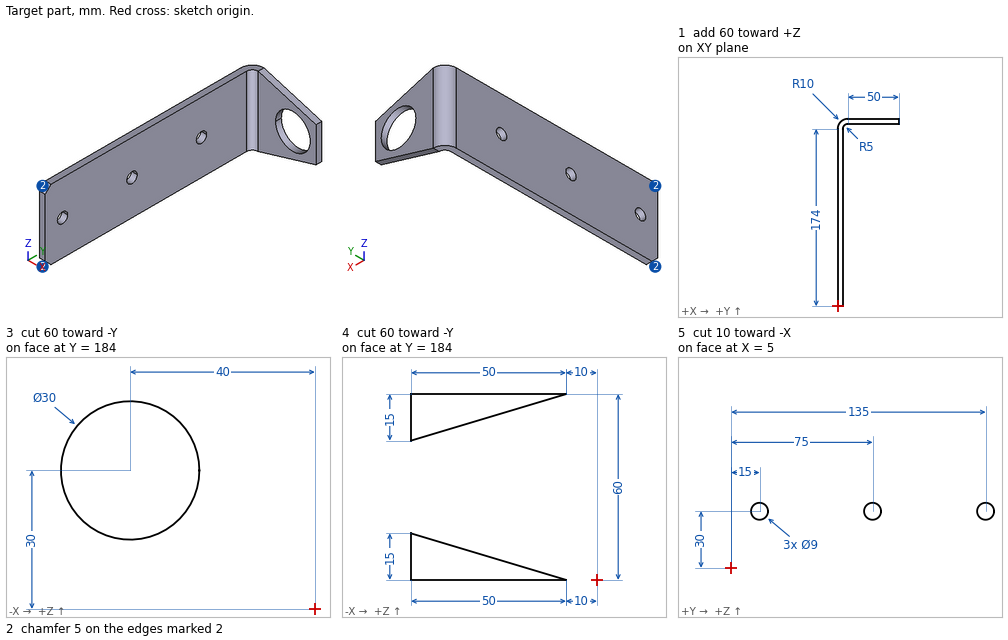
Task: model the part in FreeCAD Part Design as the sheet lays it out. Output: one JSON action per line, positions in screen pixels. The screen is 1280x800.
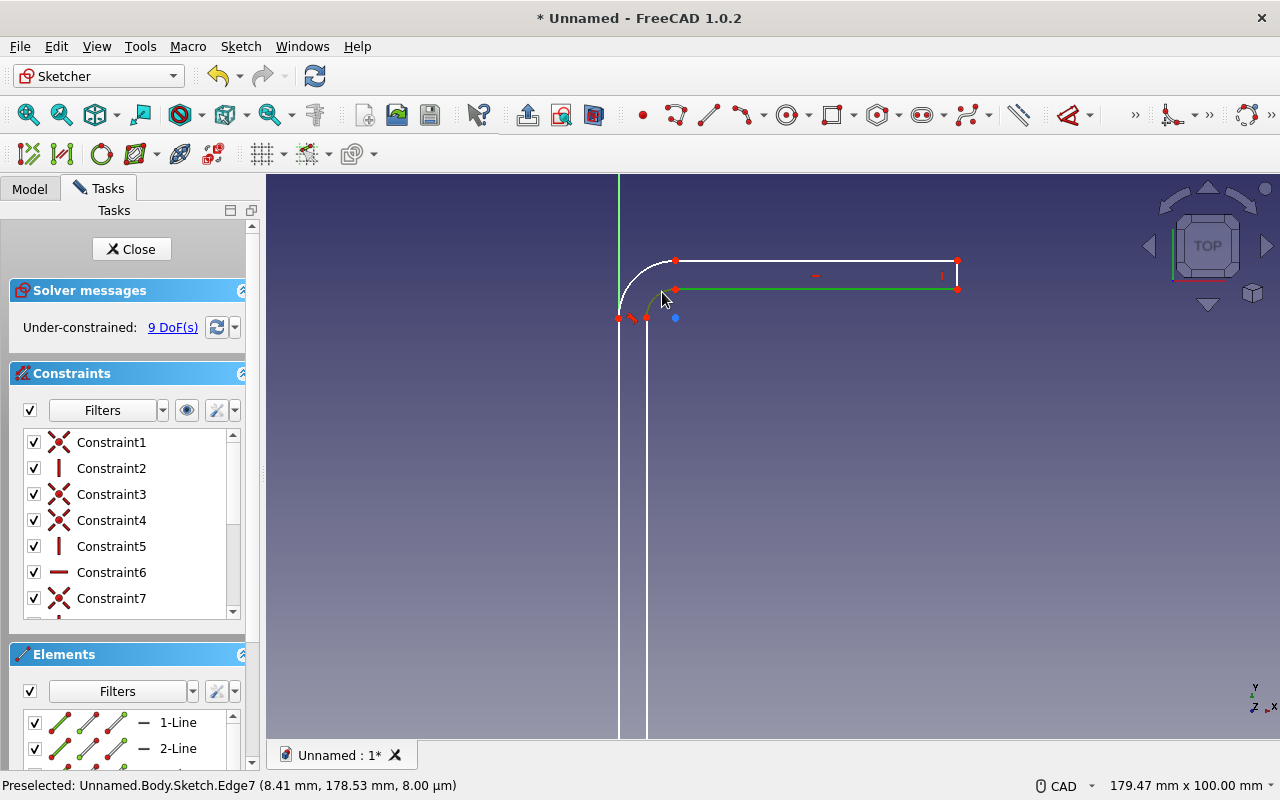
{"action": "key", "text": "t"}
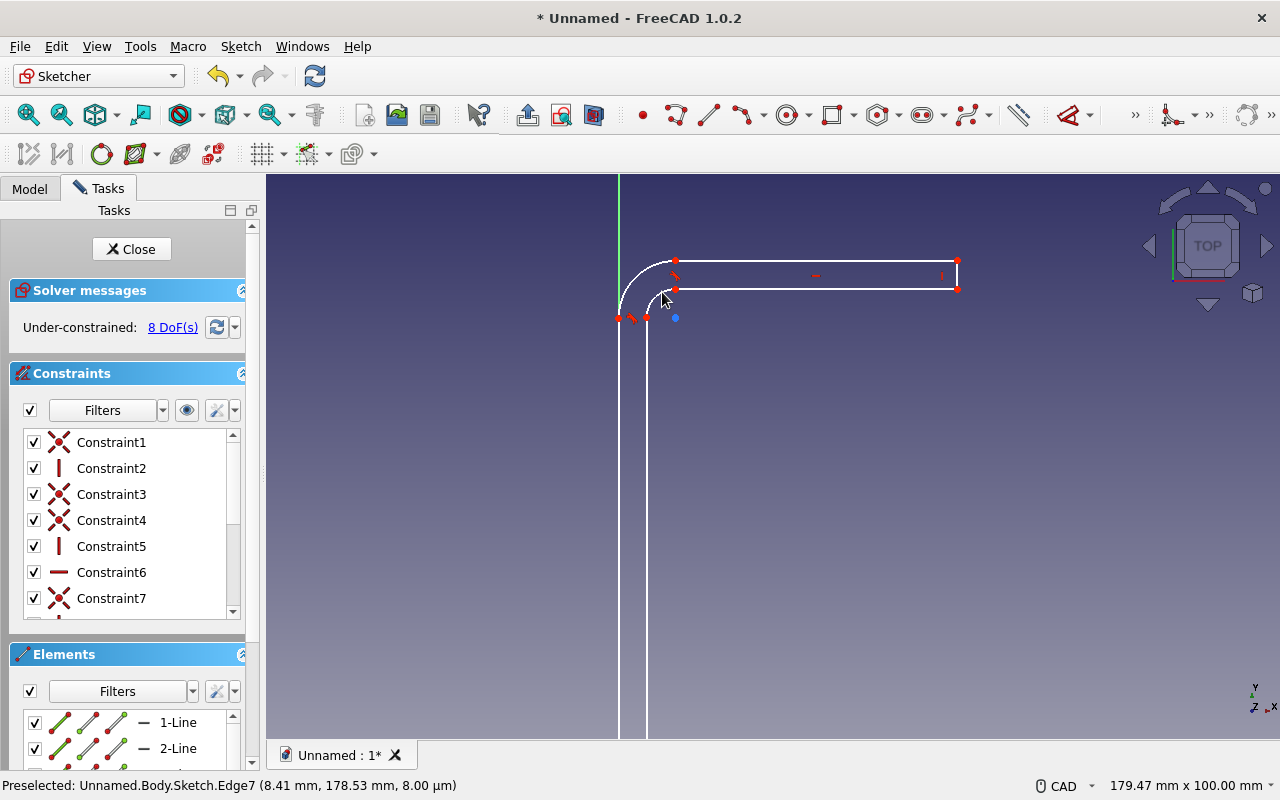
{"action": "left_click", "coordinate": [872, 261]}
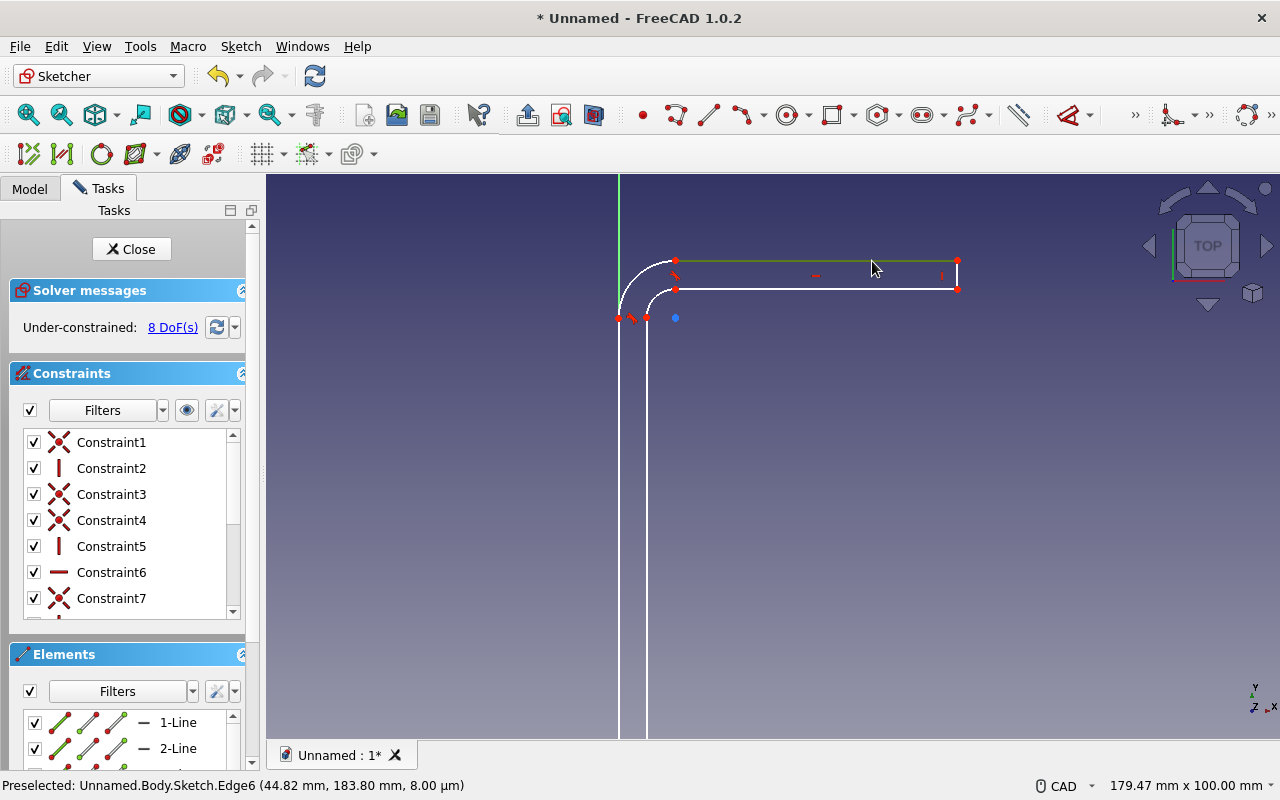
{"action": "left_click", "coordinate": [649, 267]}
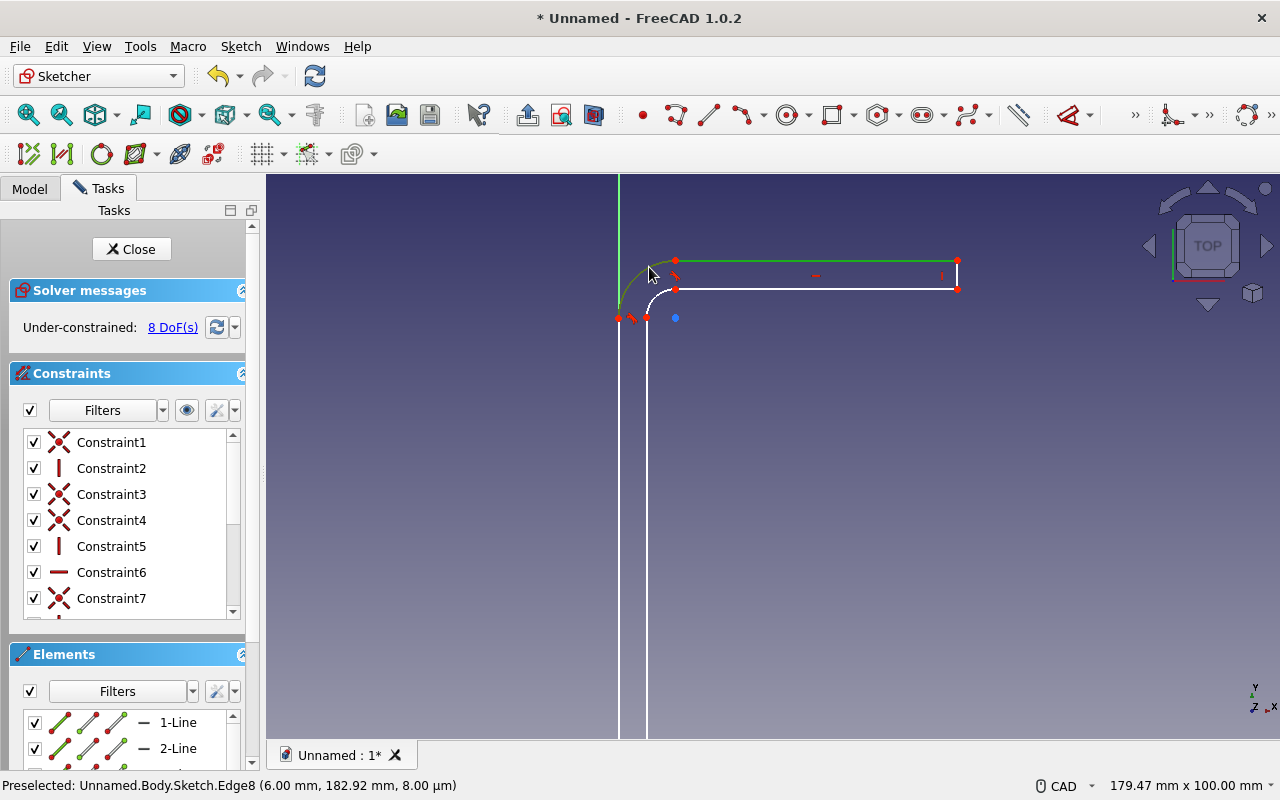
{"action": "key", "text": "t"}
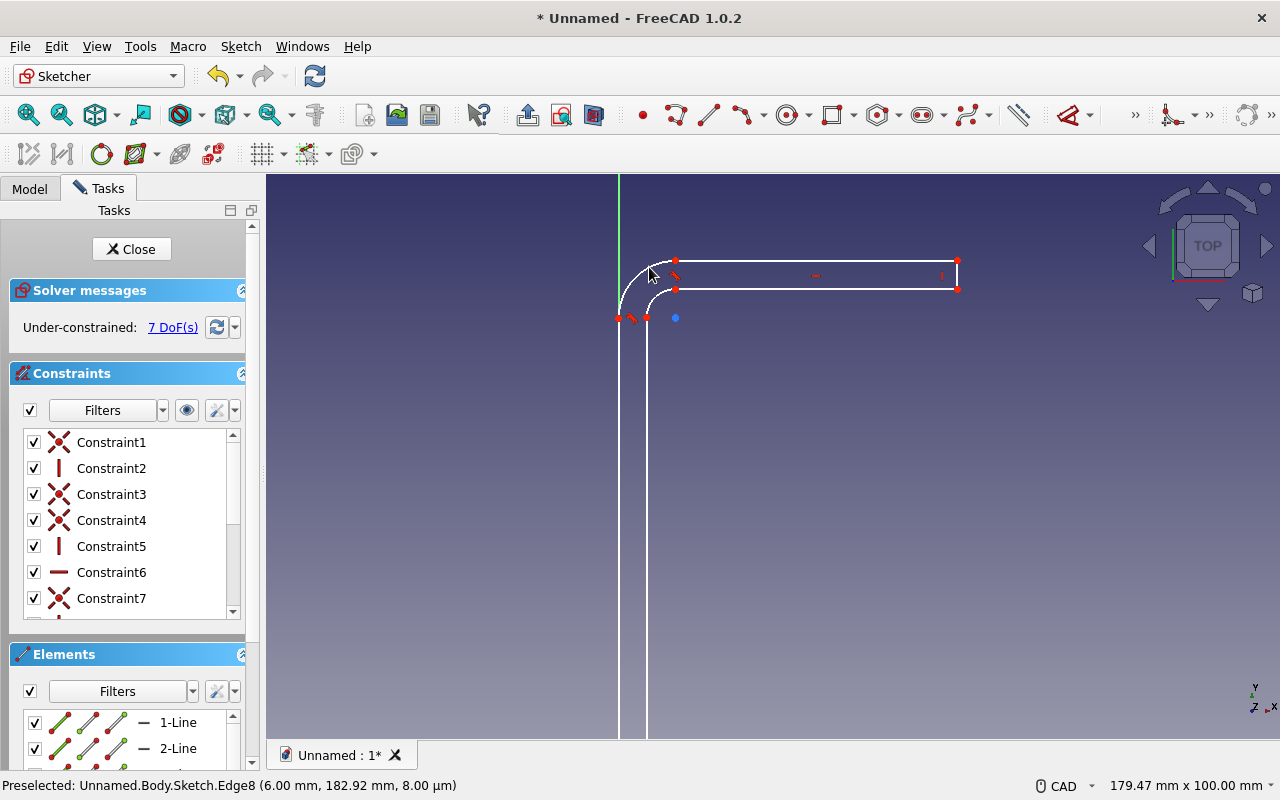
{"action": "scroll", "coordinate": [656, 269], "scroll_direction": "down", "scroll_amount": 5}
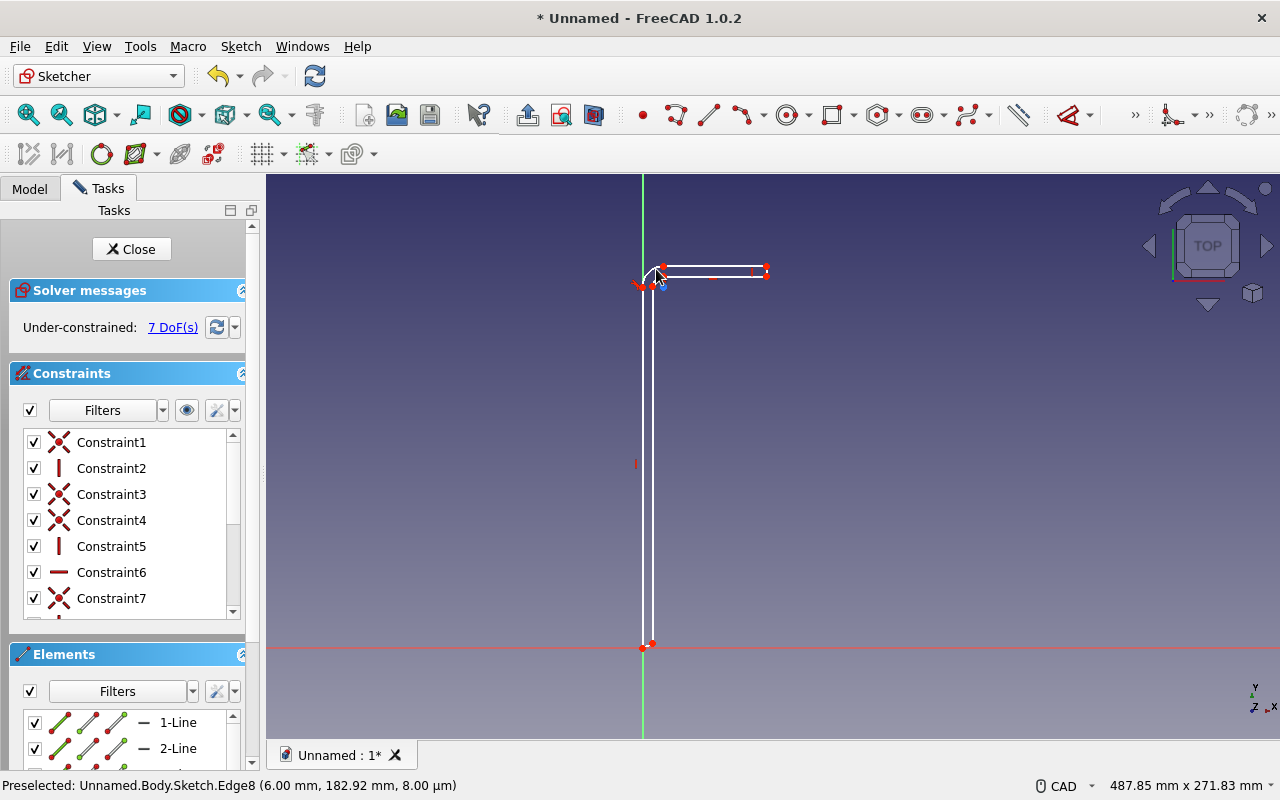
{"action": "scroll", "coordinate": [650, 645], "scroll_direction": "up", "scroll_amount": 8}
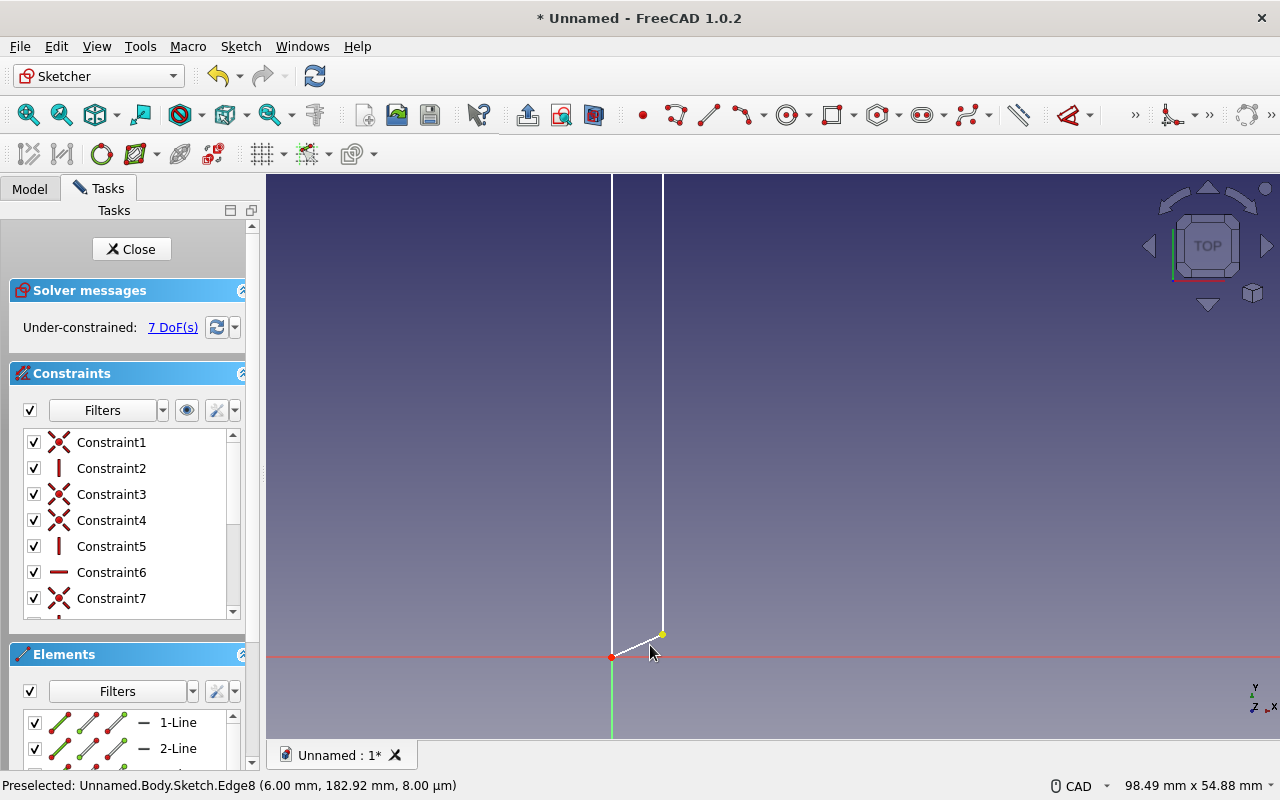
{"action": "left_click", "coordinate": [647, 641]}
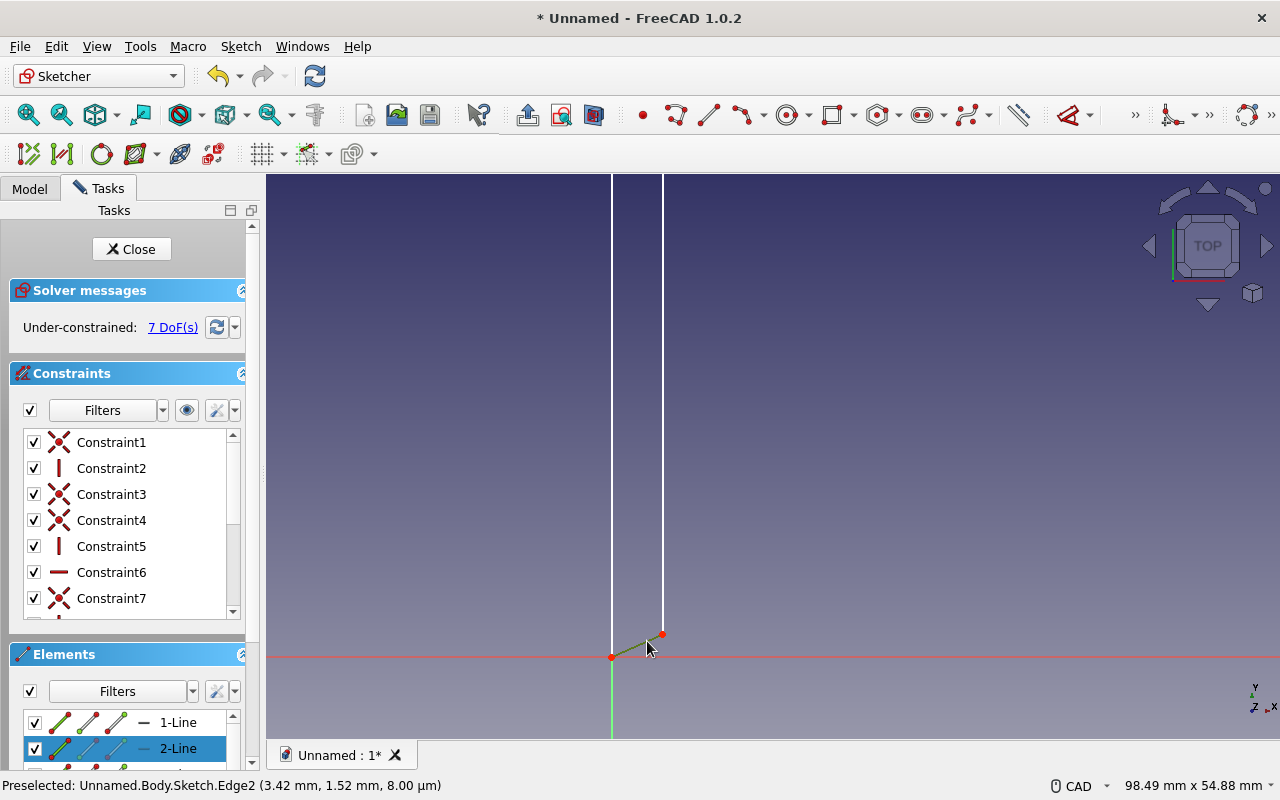
{"action": "key", "text": "h"}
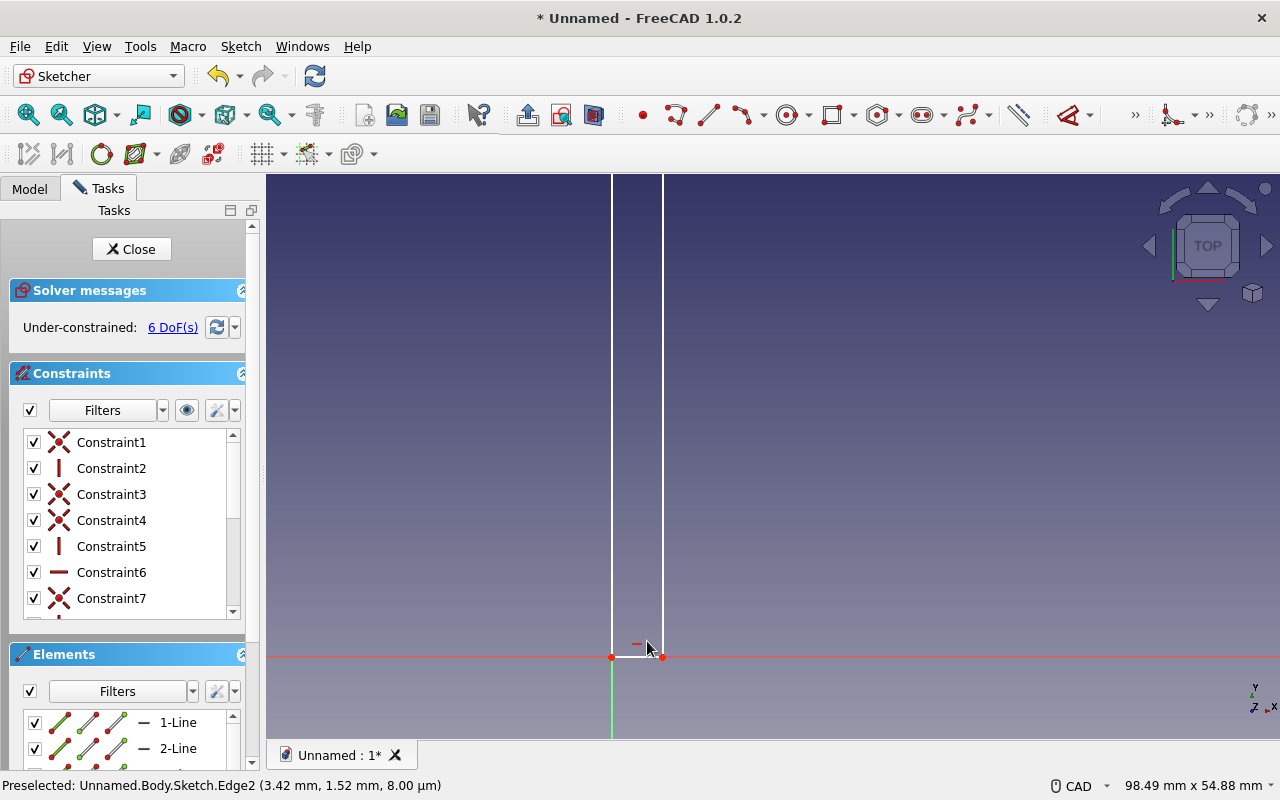
{"action": "scroll", "coordinate": [650, 645], "scroll_direction": "down", "scroll_amount": 8}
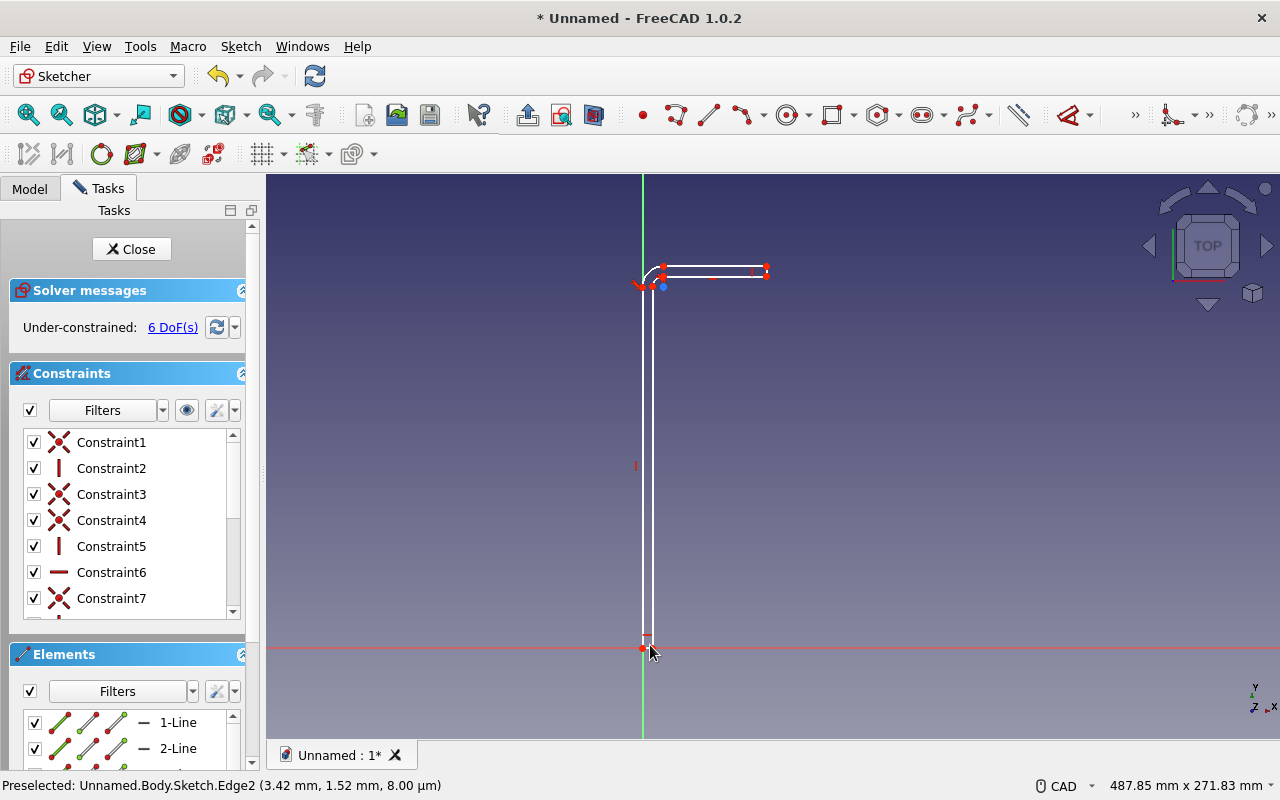
{"action": "scroll", "coordinate": [659, 278], "scroll_direction": "up", "scroll_amount": 6}